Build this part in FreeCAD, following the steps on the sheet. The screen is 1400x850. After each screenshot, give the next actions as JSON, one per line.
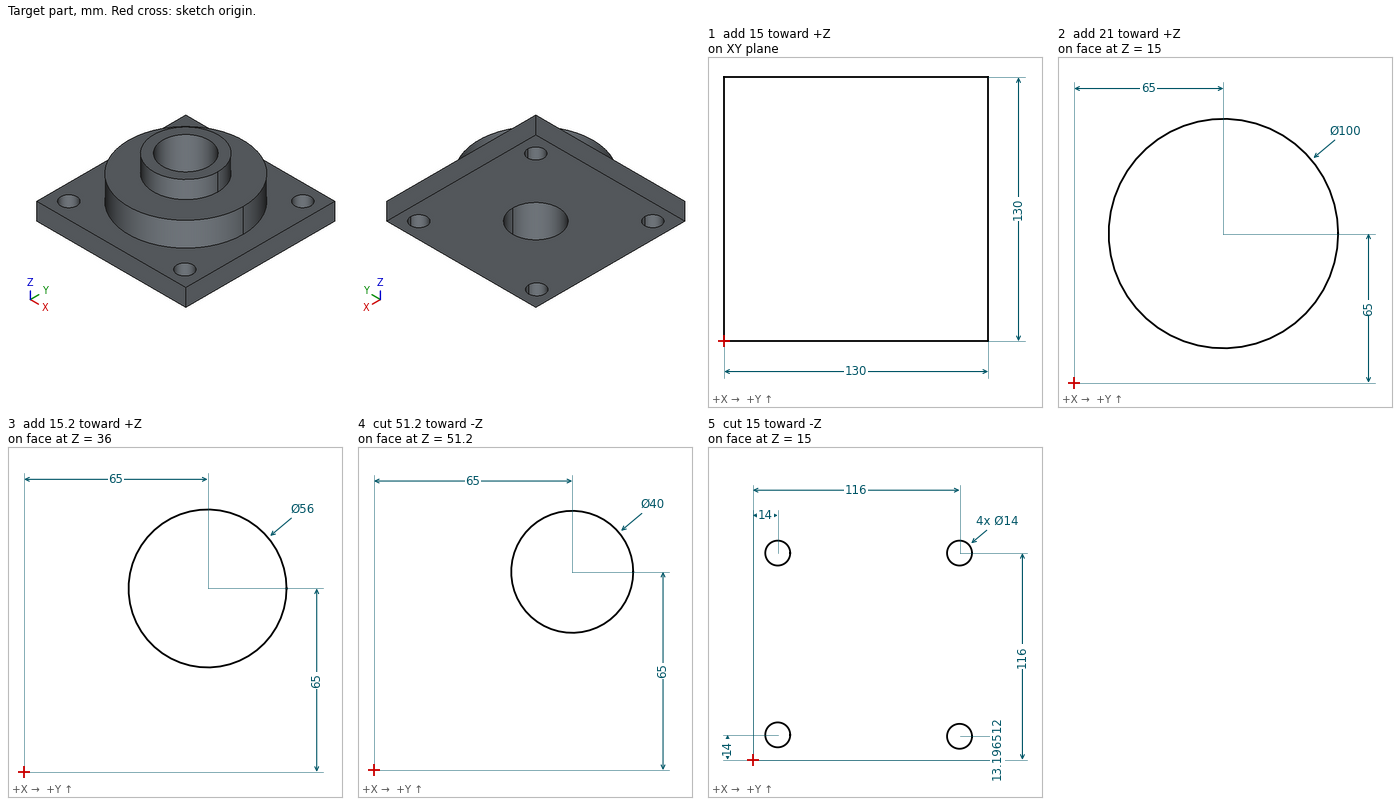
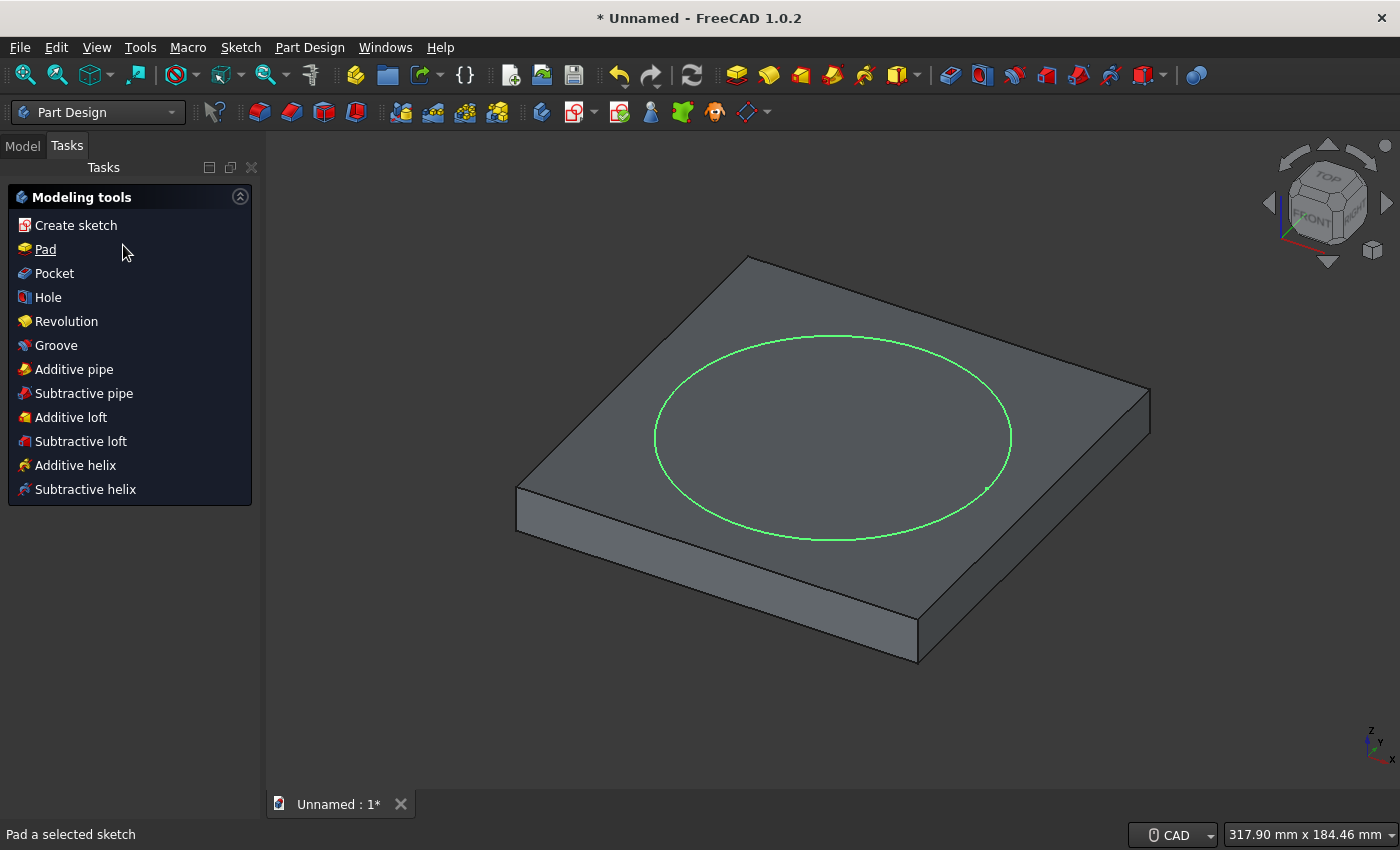
{"action": "left_click", "coordinate": [738, 76]}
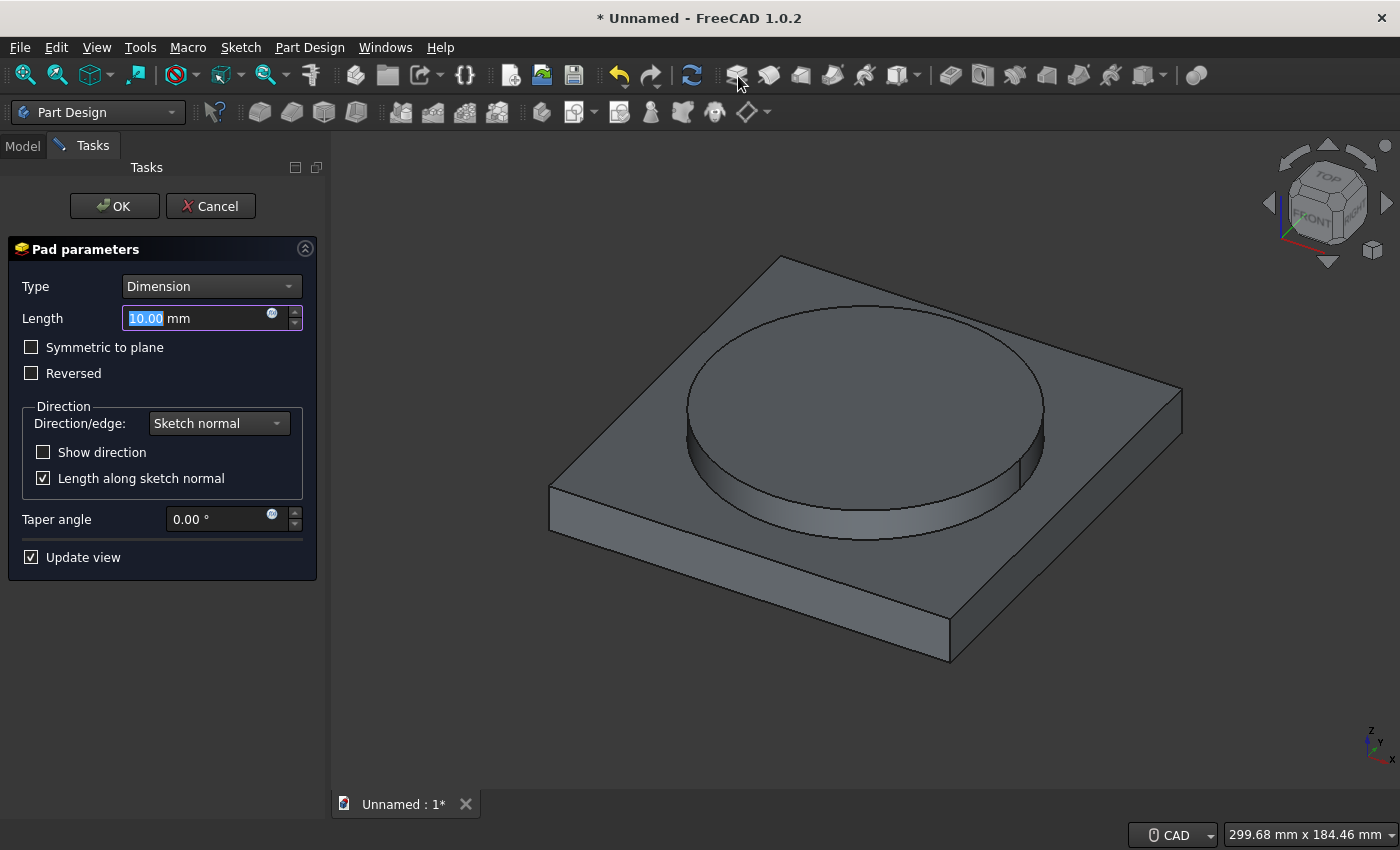
{"action": "type", "text": "21"}
{"action": "key", "text": "Tab"}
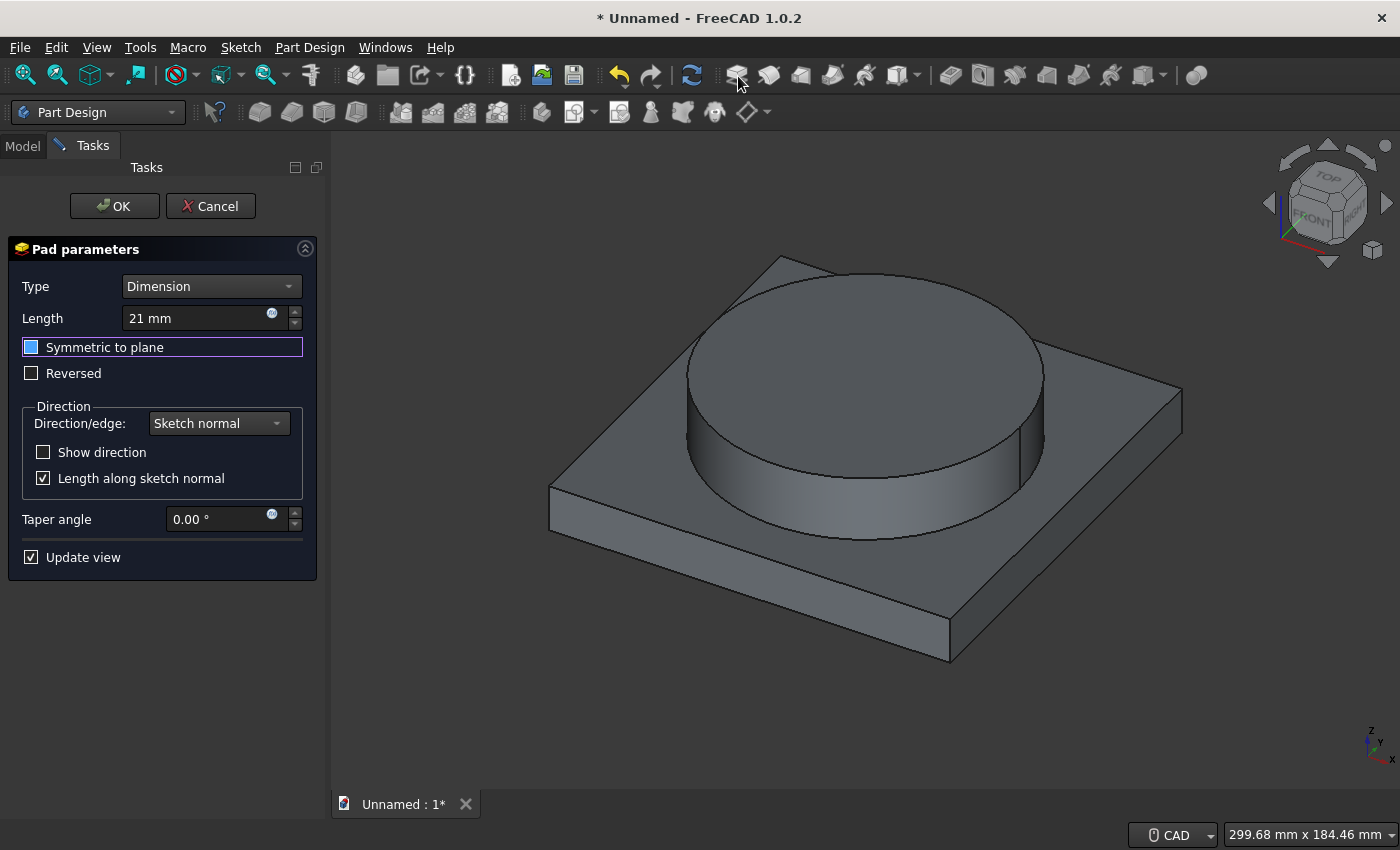
{"action": "left_click", "coordinate": [115, 206]}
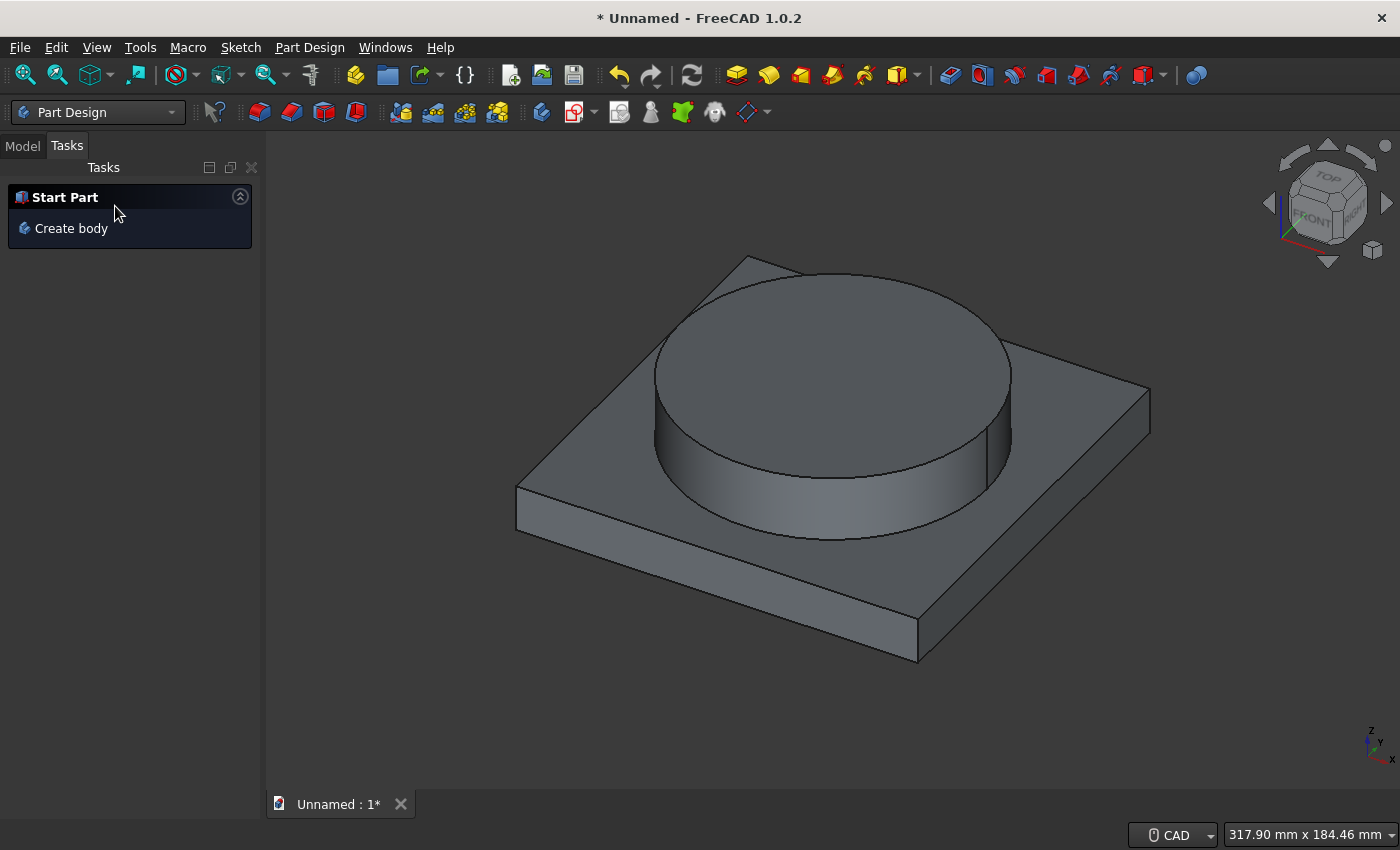
{"action": "left_click", "coordinate": [833, 375]}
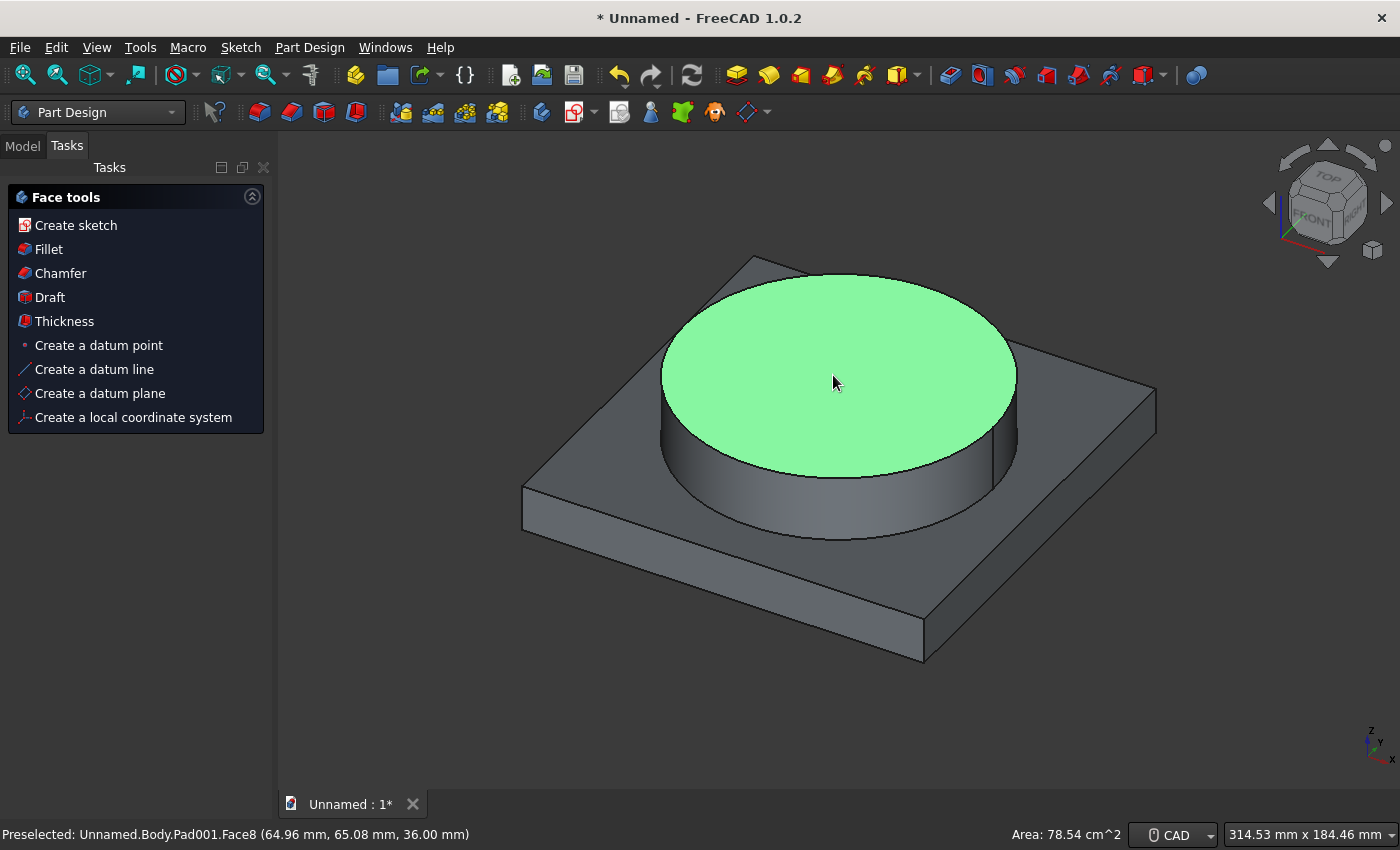
{"action": "left_click", "coordinate": [574, 112]}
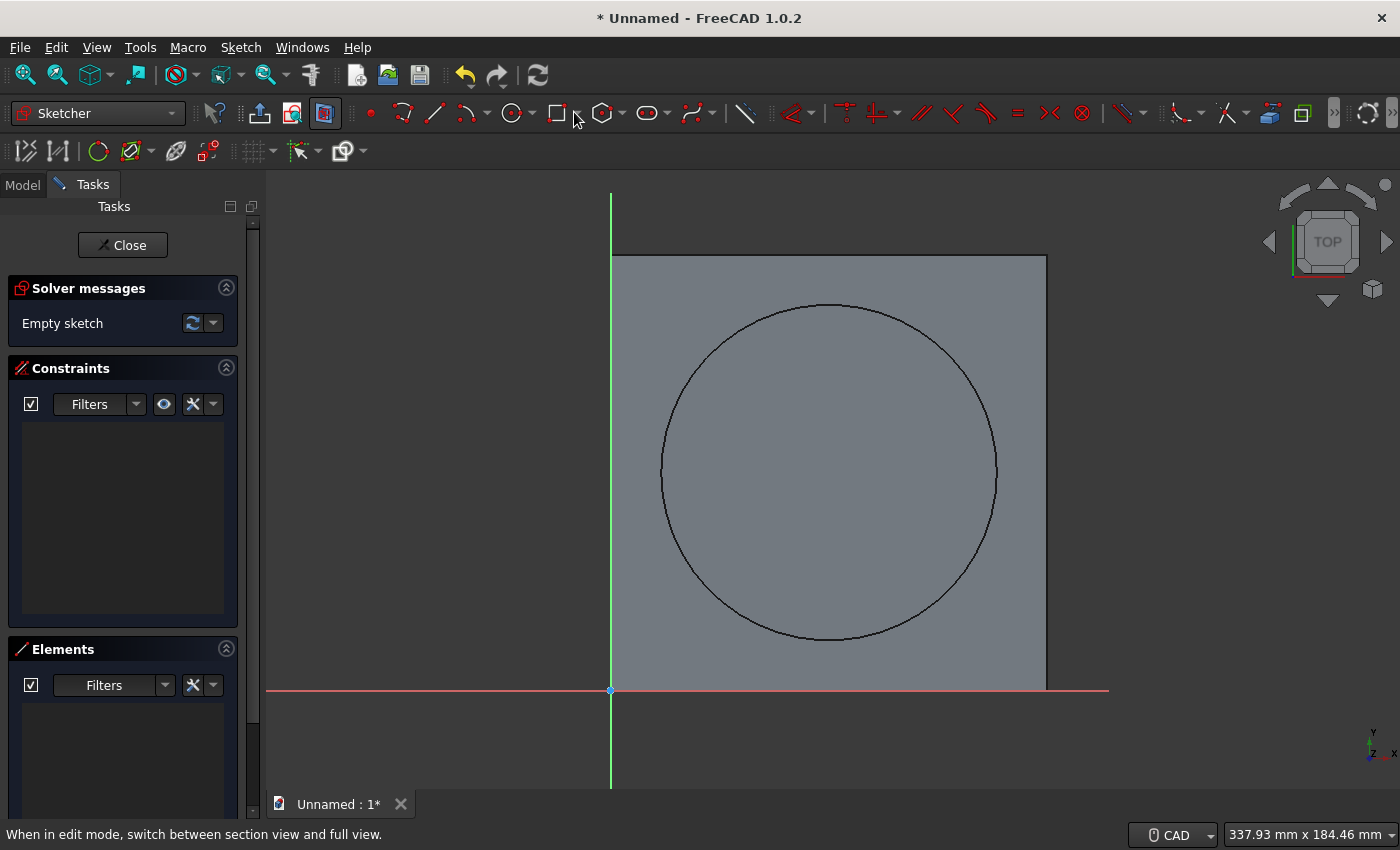
{"action": "key", "text": "g c"}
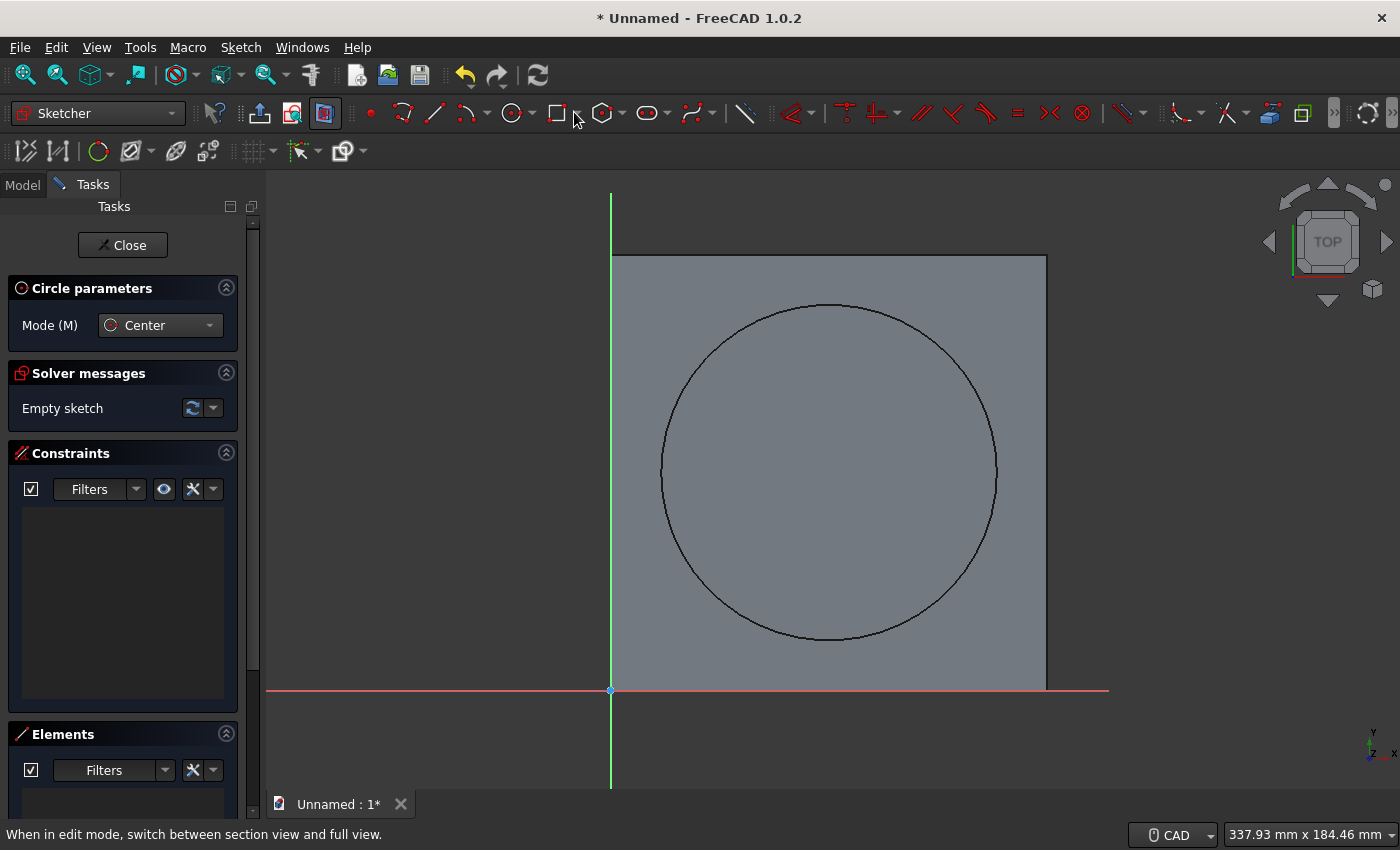
{"action": "left_click", "coordinate": [829, 473]}
{"action": "mouse_move", "coordinate": [895, 406]}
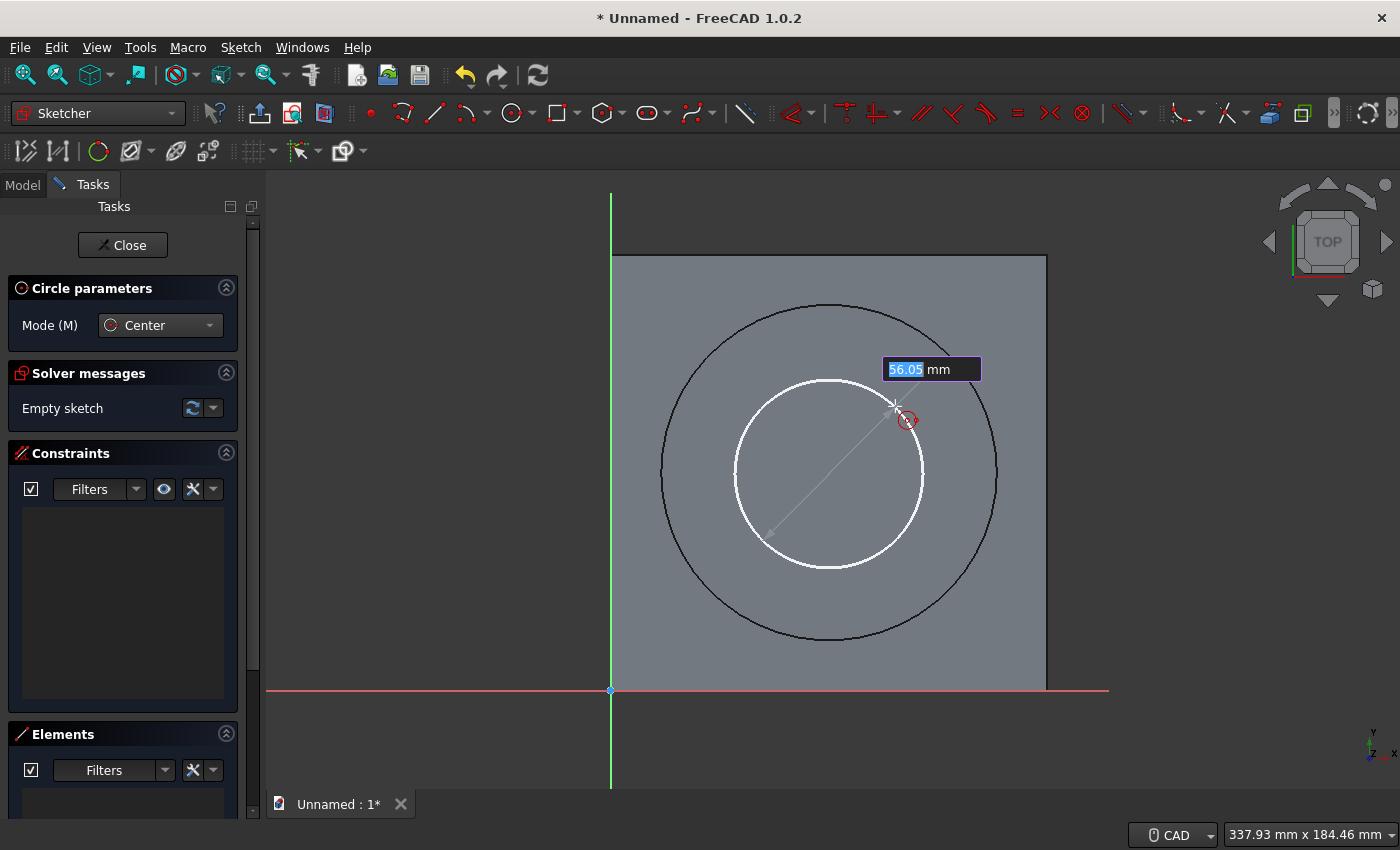
{"action": "type", "text": "56"}
{"action": "key", "text": "Return"}
{"action": "key", "text": "Escape"}